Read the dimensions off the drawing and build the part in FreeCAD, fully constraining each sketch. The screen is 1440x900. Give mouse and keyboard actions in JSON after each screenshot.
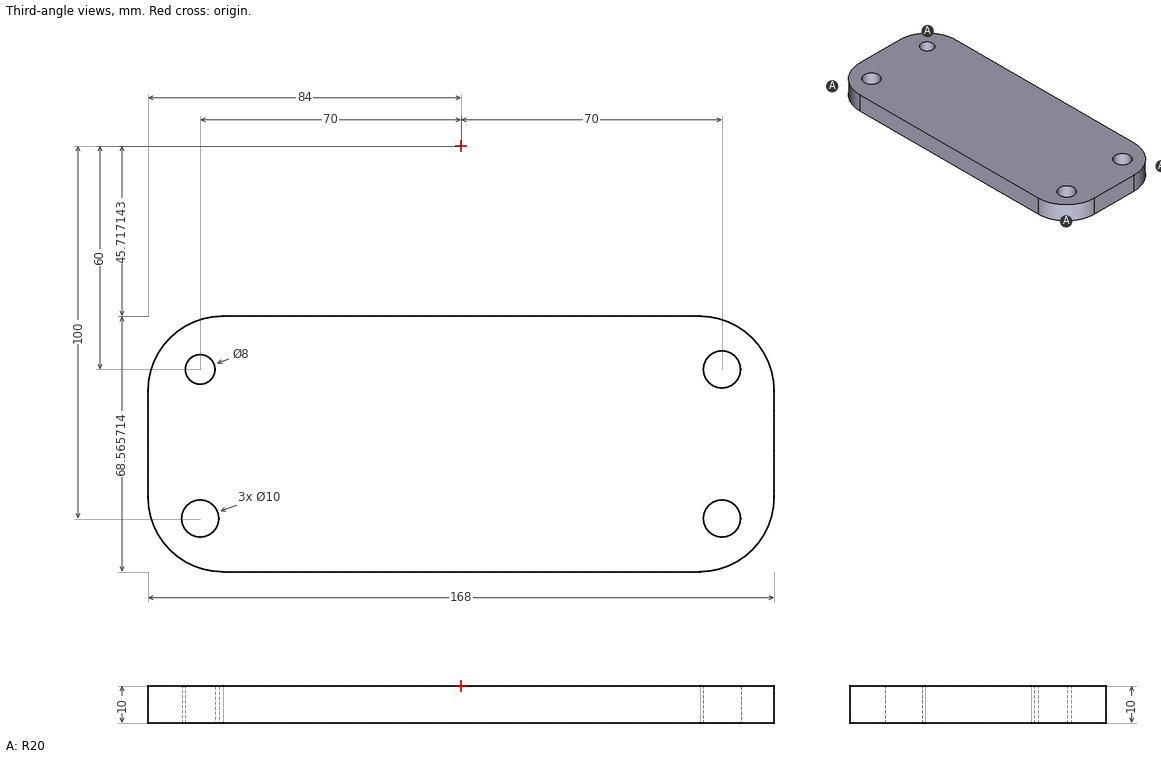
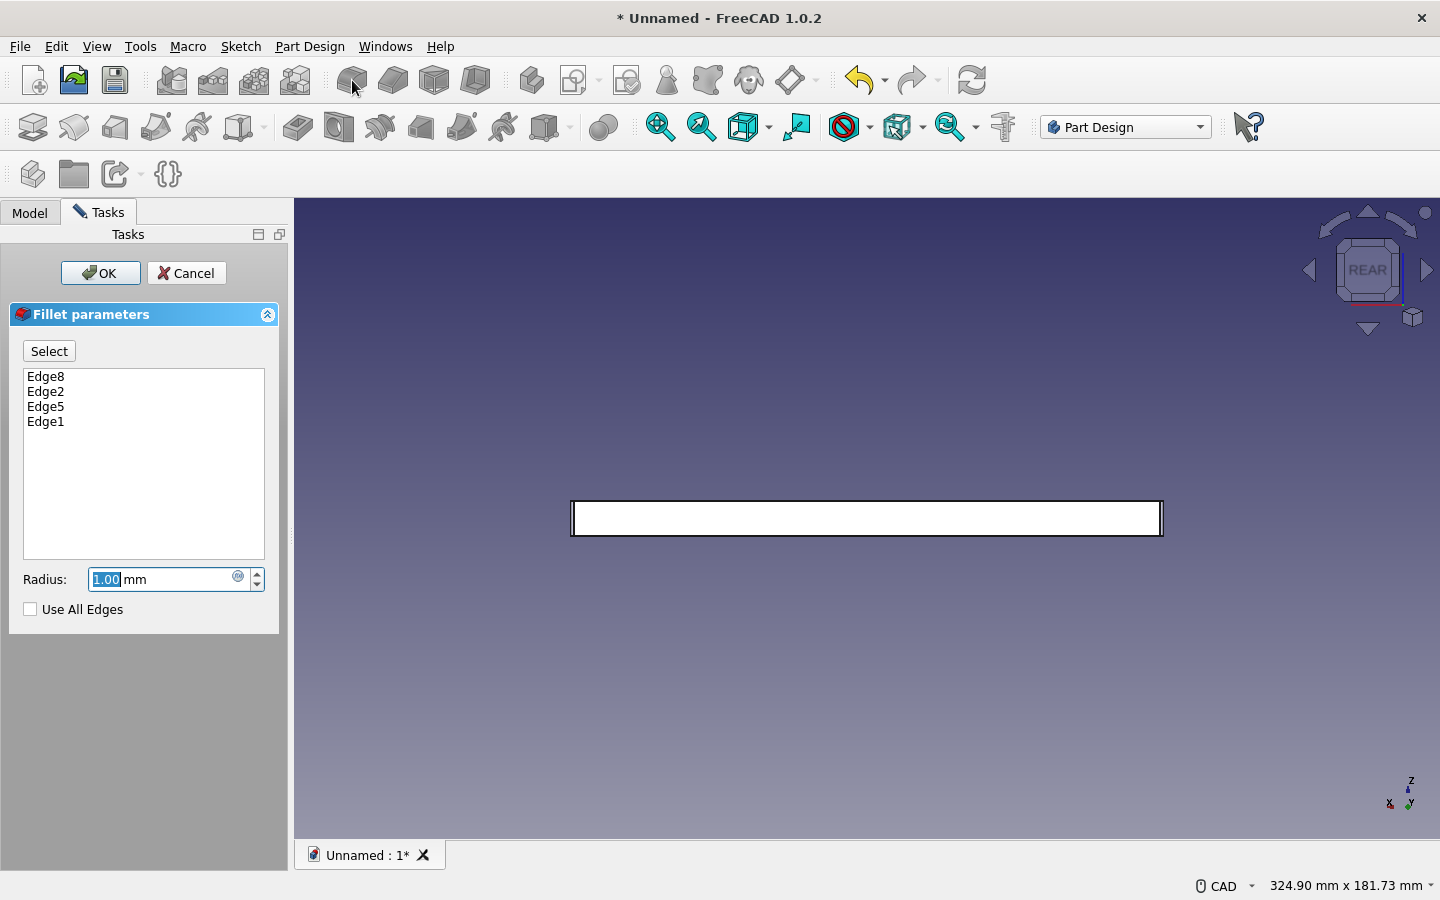
{"action": "type", "text": "20"}
{"action": "key", "text": "Tab"}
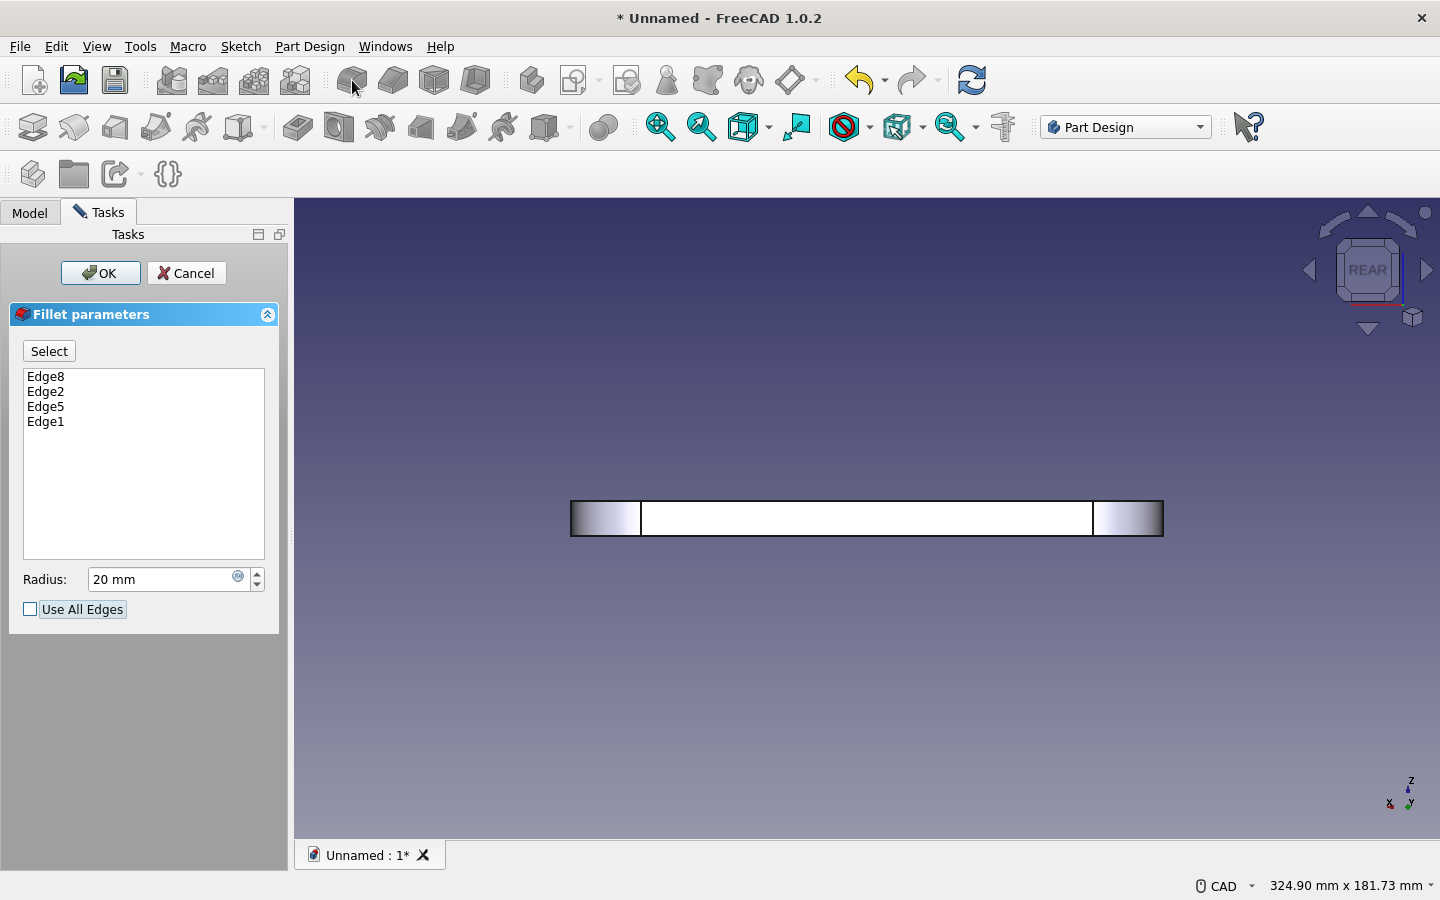
{"action": "left_click", "coordinate": [101, 273]}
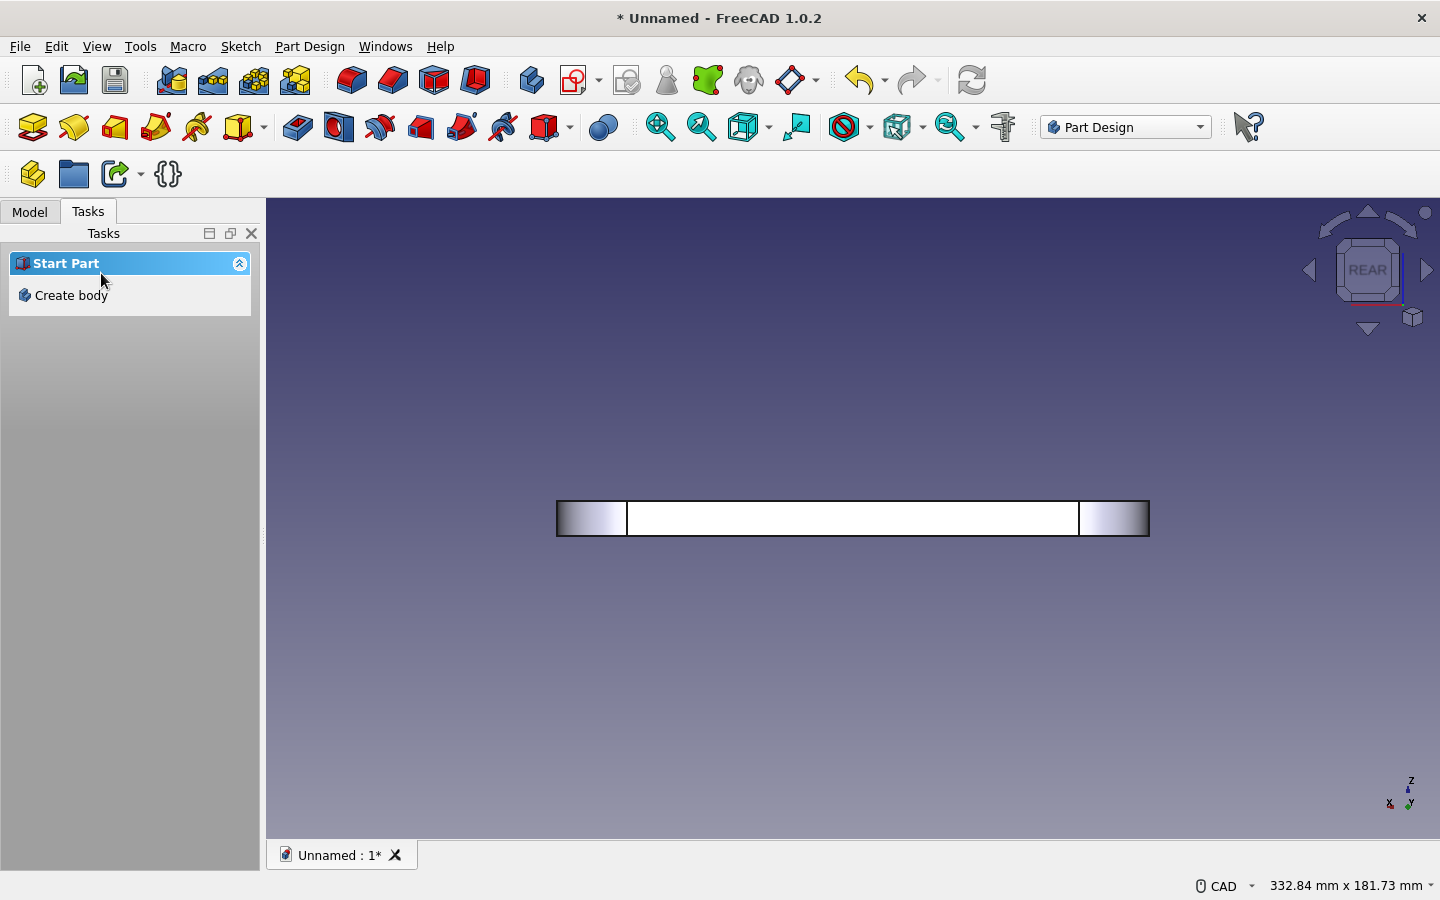
{"action": "key", "text": "0"}